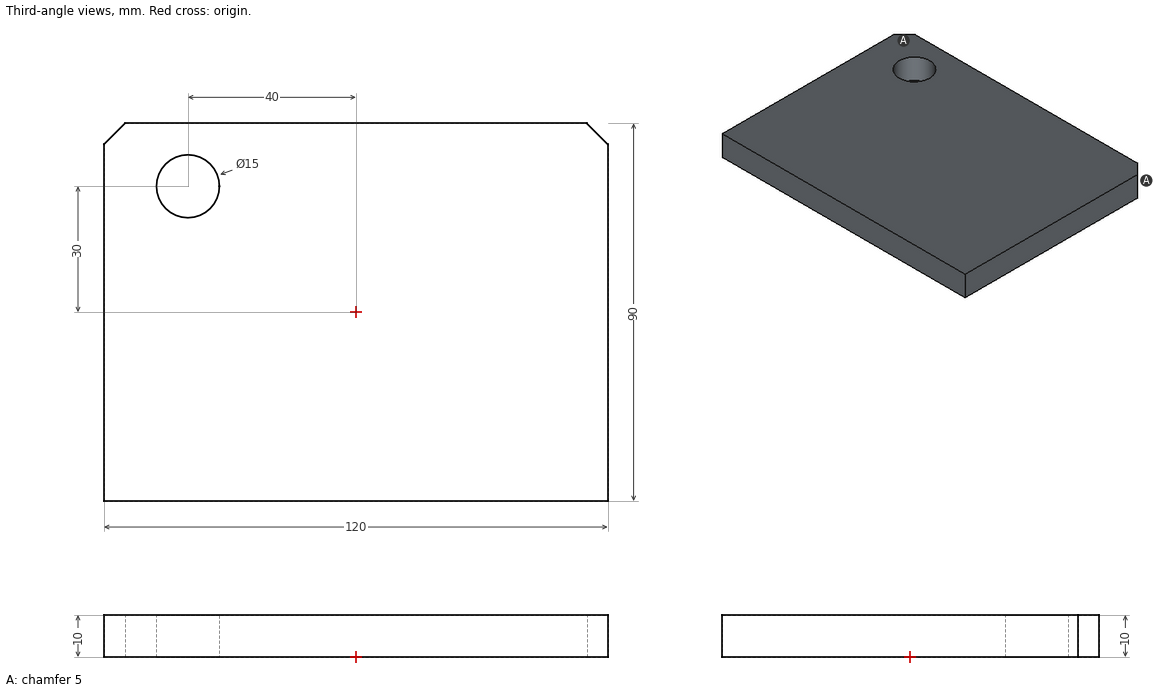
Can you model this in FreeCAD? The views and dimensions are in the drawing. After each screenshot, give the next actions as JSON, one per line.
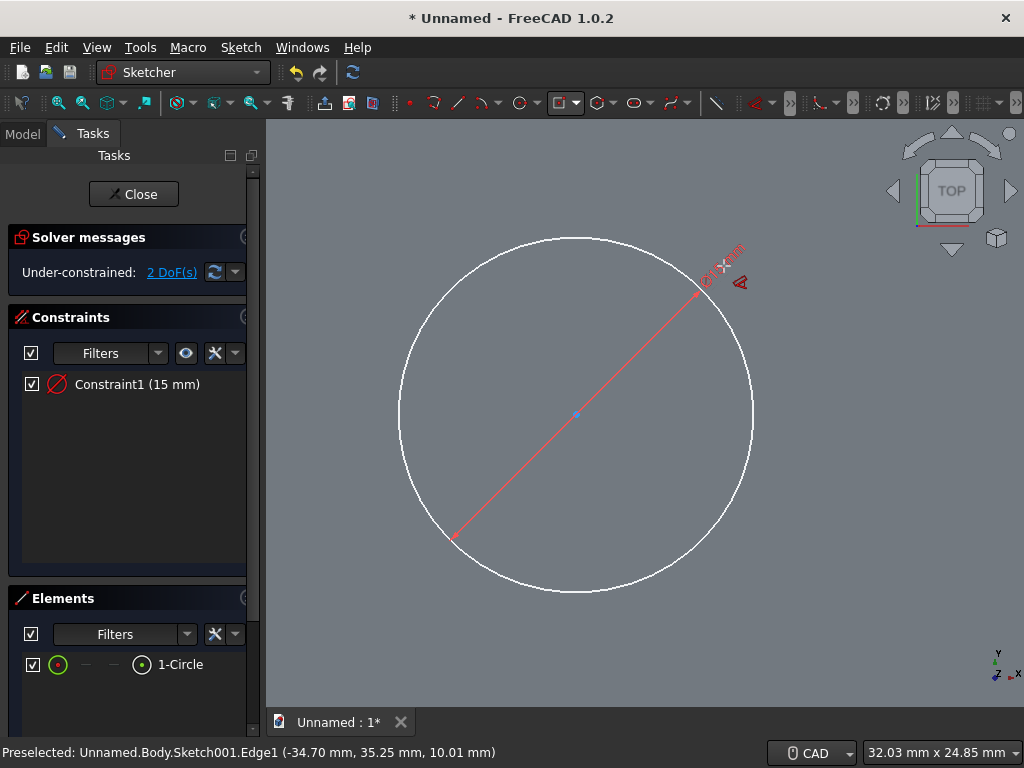
{"action": "left_click", "coordinate": [576, 415]}
{"action": "left_click", "coordinate": [717, 381]}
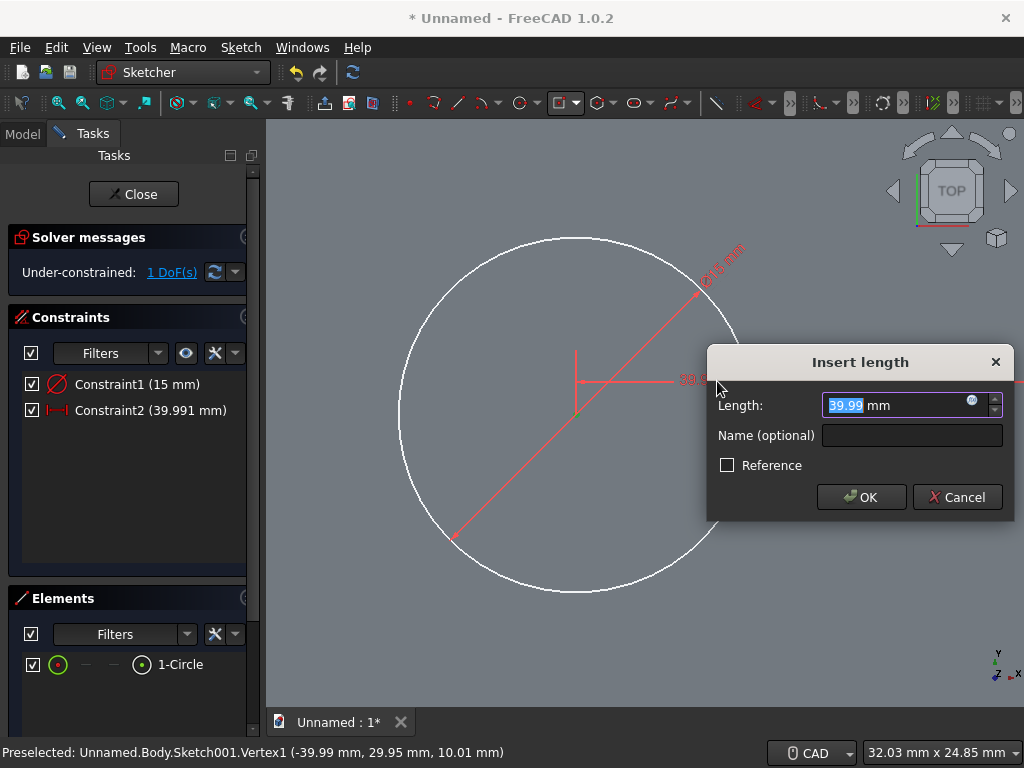
{"action": "type", "text": "40"}
{"action": "key", "text": "Return"}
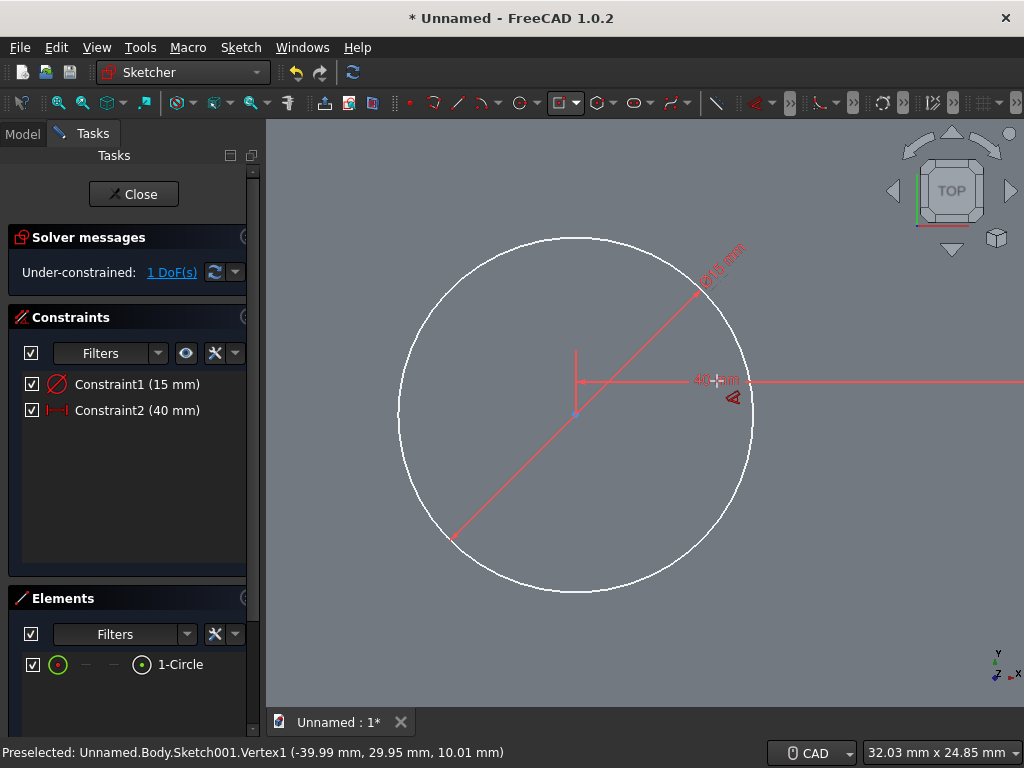
{"action": "left_click", "coordinate": [576, 415]}
{"action": "left_click", "coordinate": [542, 547]}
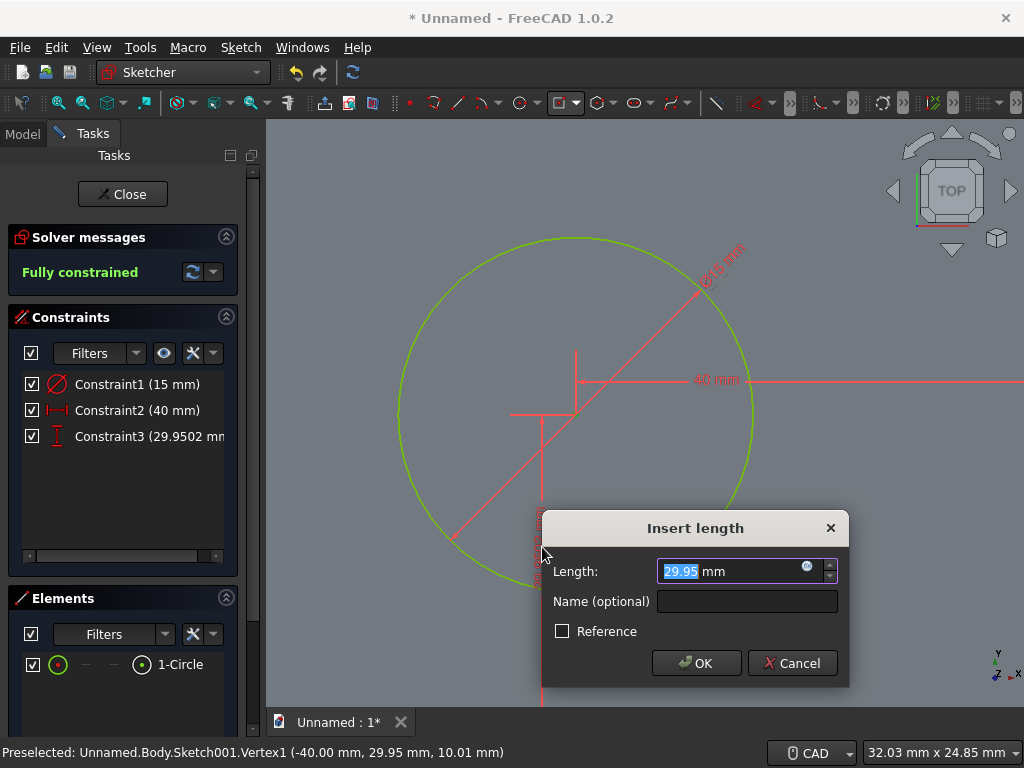
{"action": "type", "text": "30"}
{"action": "key", "text": "Return"}
{"action": "key", "text": "Escape"}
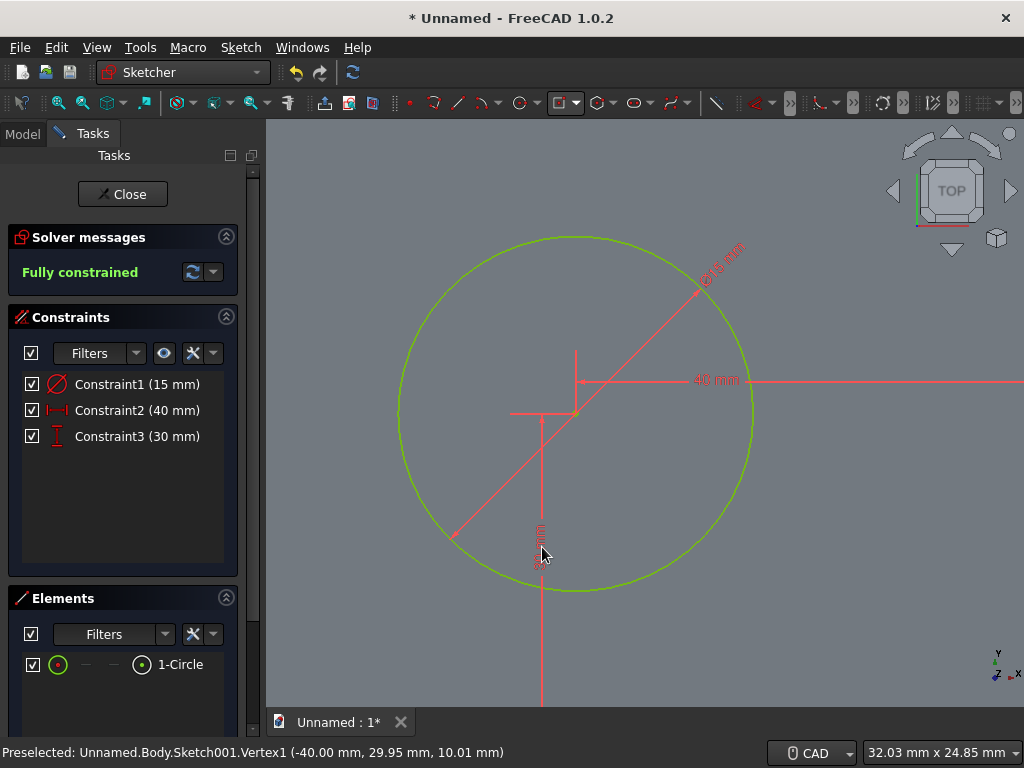
{"action": "left_click", "coordinate": [123, 194]}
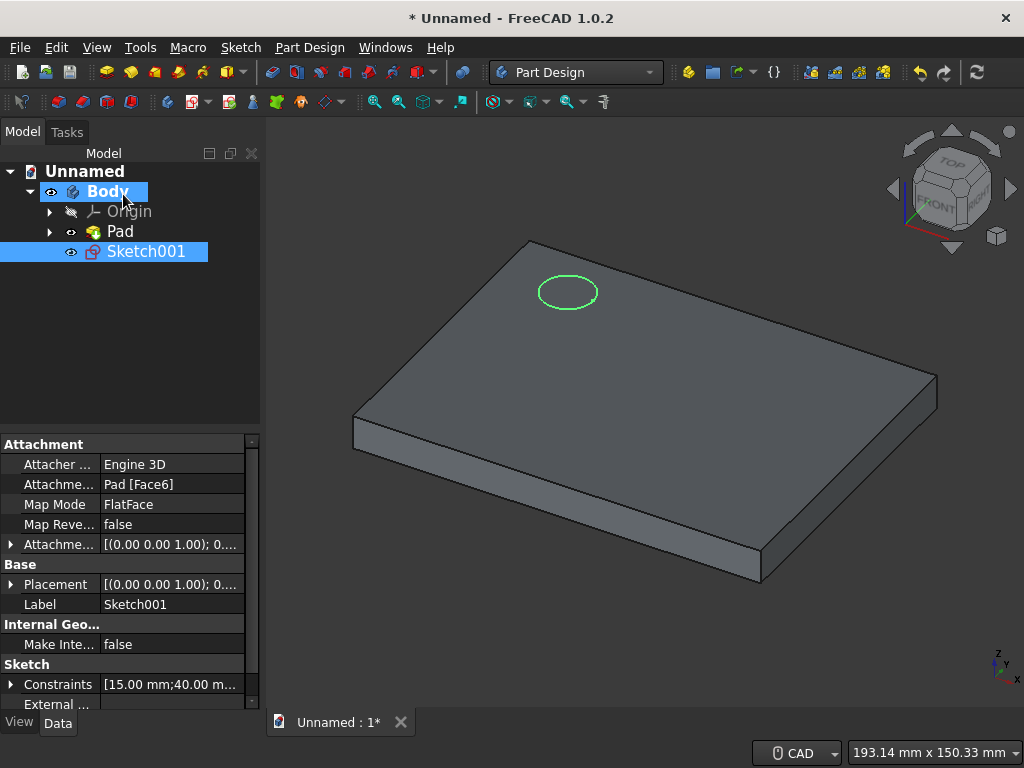
{"action": "left_click", "coordinate": [274, 72]}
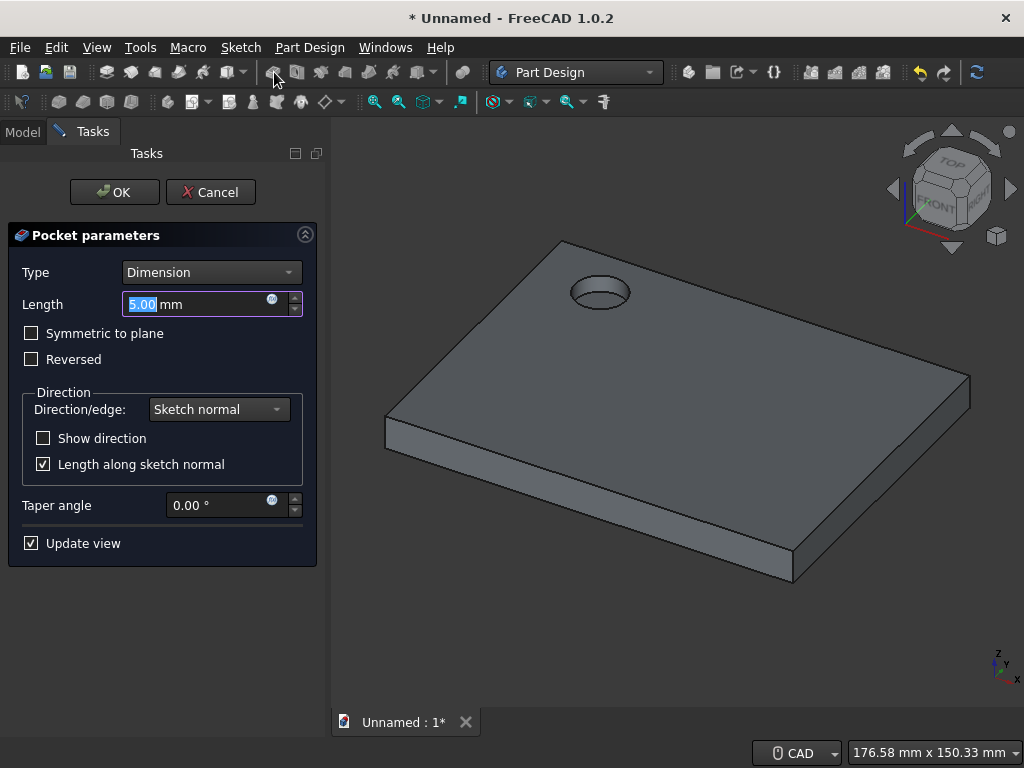
{"action": "type", "text": "10"}
{"action": "key", "text": "Tab"}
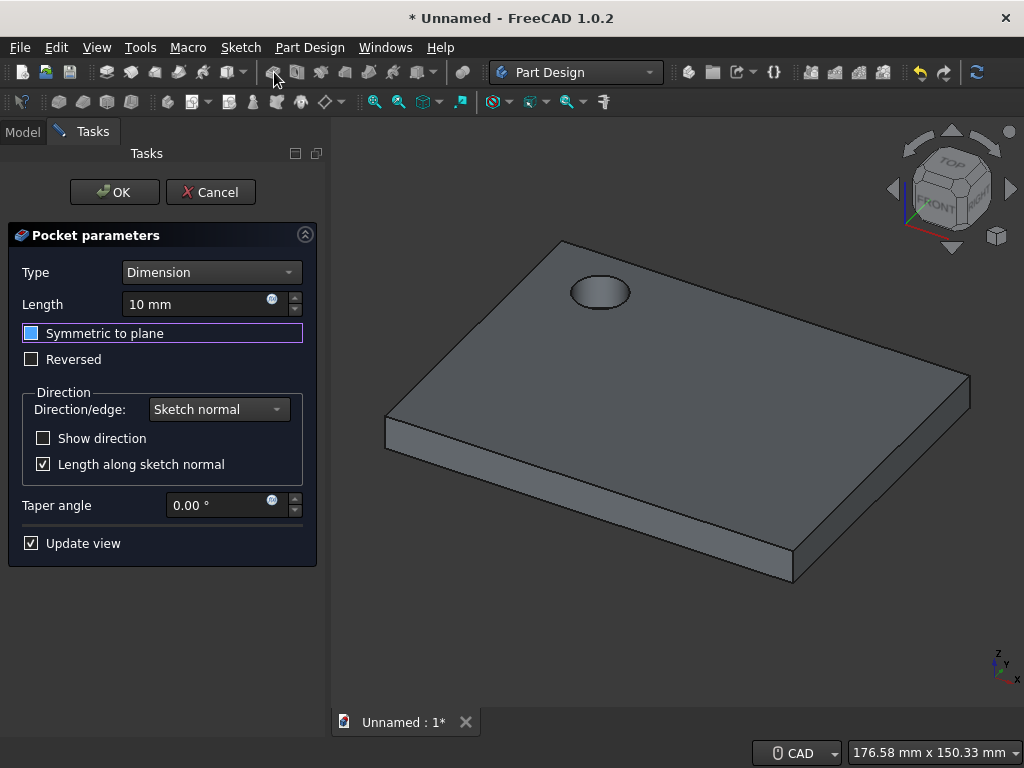
{"action": "left_click", "coordinate": [115, 192]}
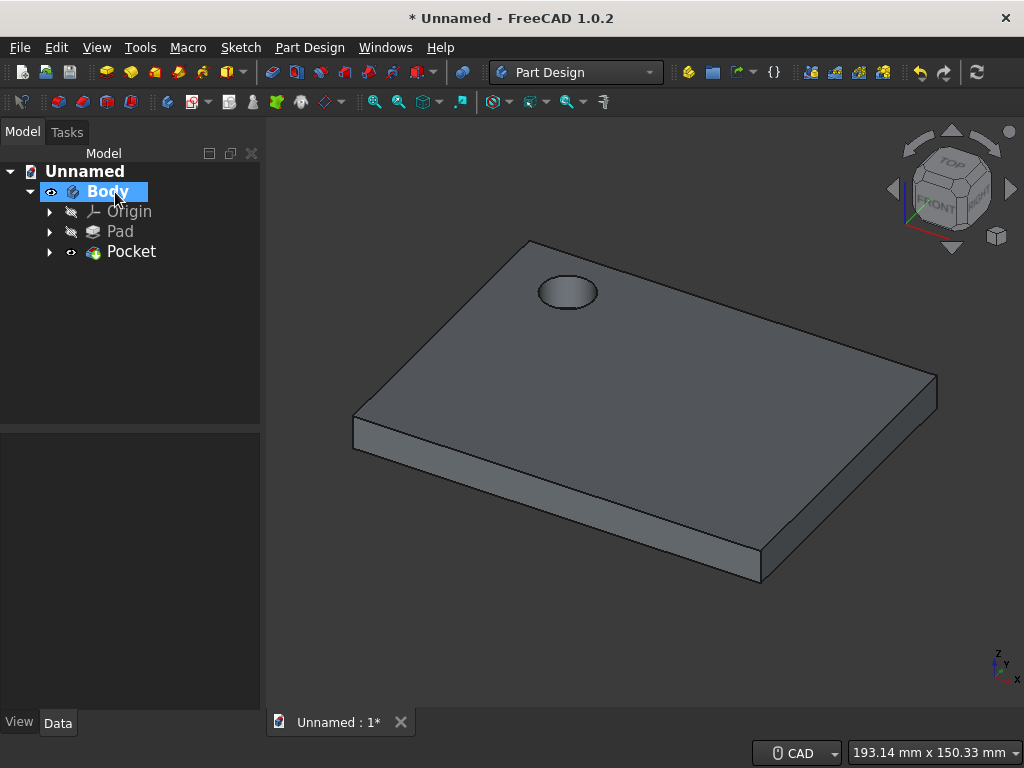
{"action": "key", "text": "0"}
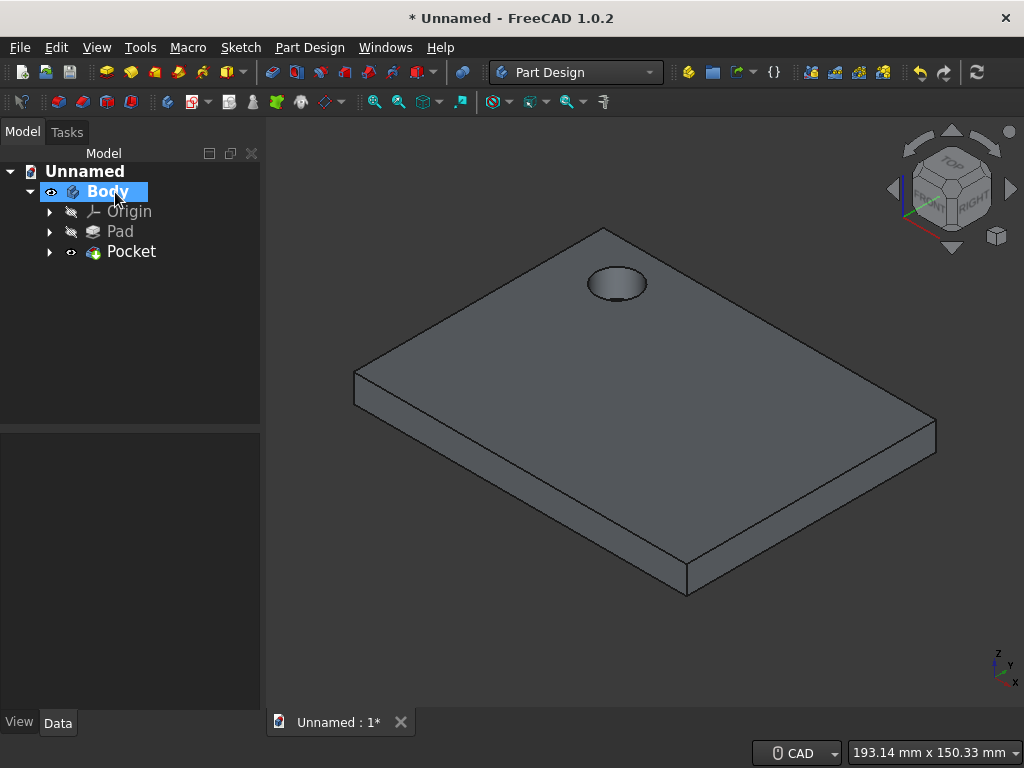
{"action": "key", "text": "2"}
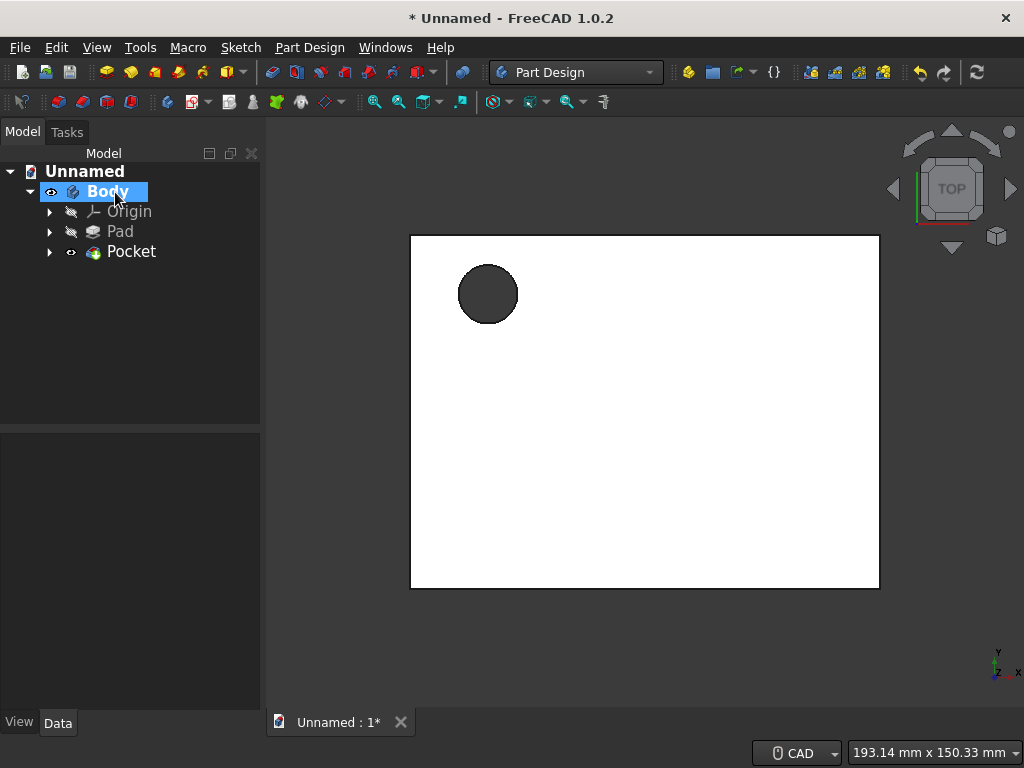
{"action": "key", "text": "1"}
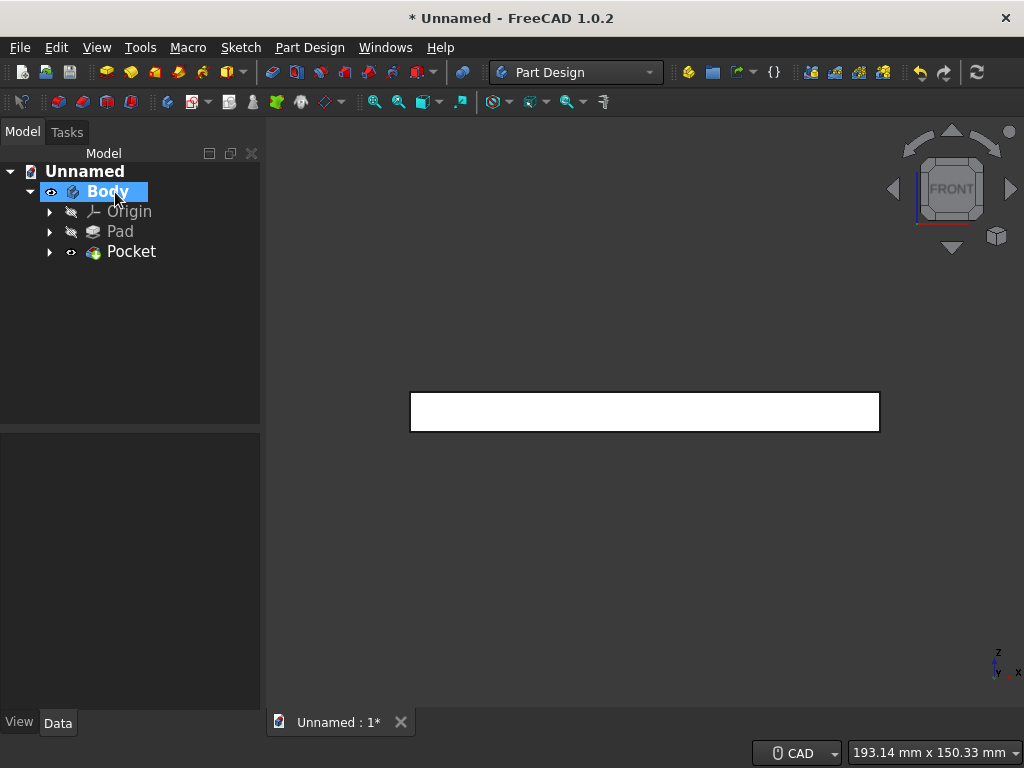
{"action": "key", "text": "3"}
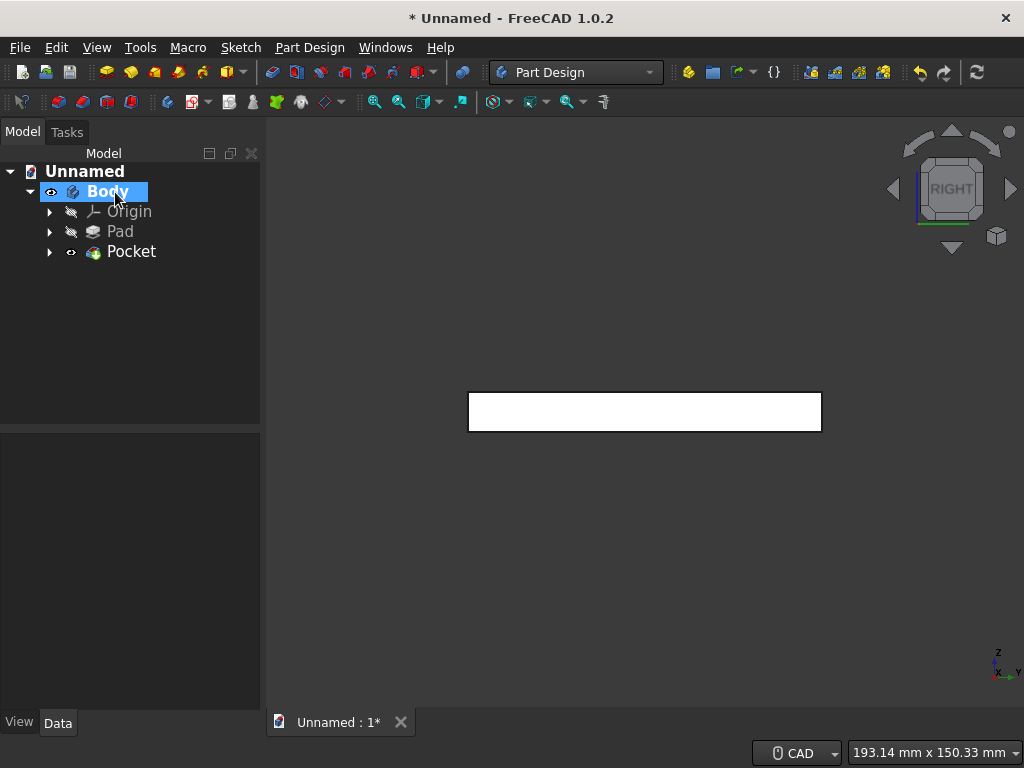
{"action": "left_click", "coordinate": [822, 411]}